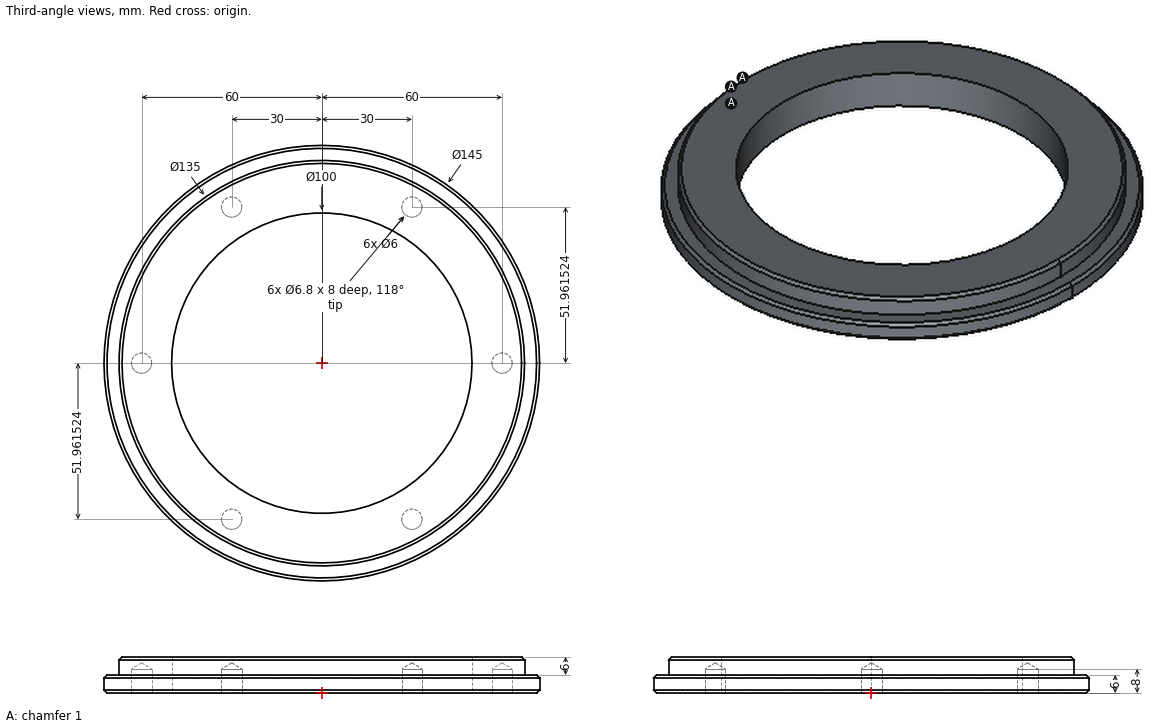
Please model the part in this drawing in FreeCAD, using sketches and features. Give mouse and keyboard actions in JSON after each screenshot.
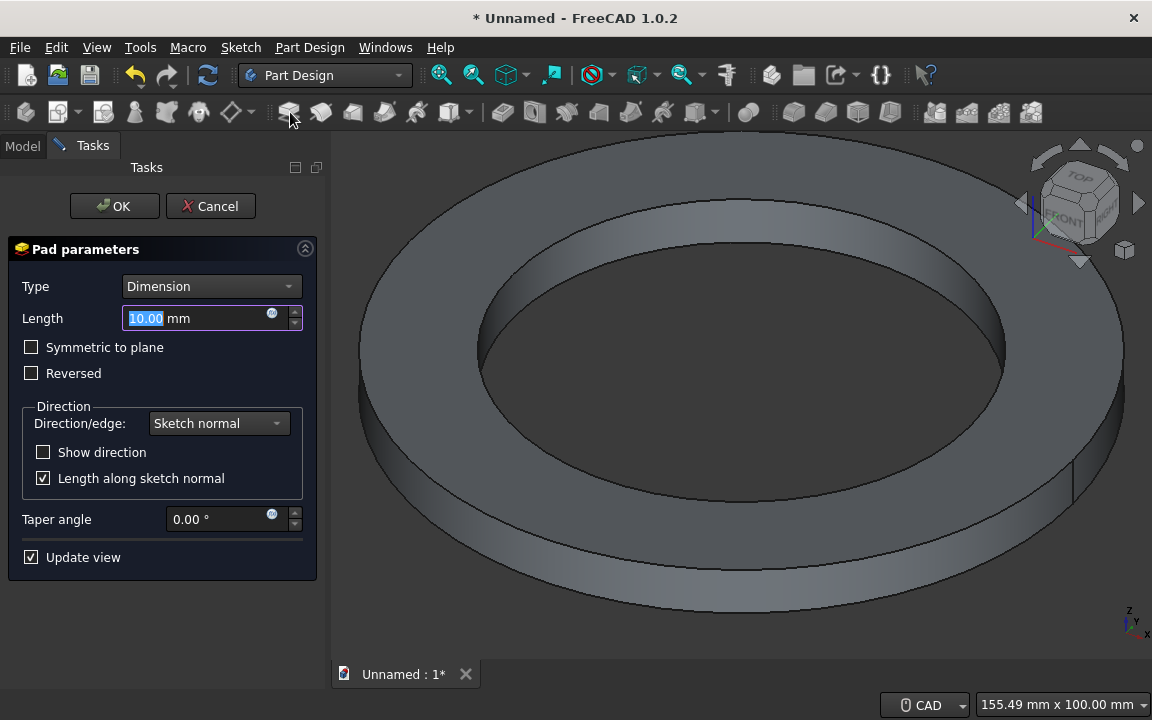
{"action": "type", "text": "6"}
{"action": "key", "text": "Tab"}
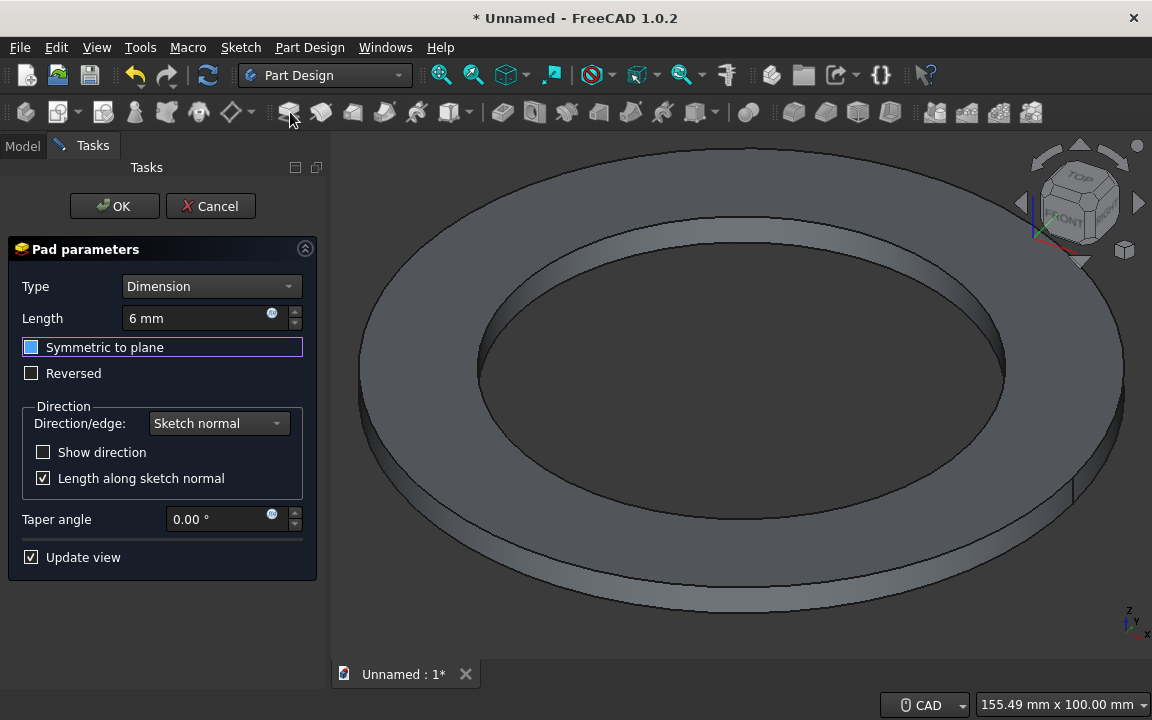
{"action": "left_click", "coordinate": [115, 206]}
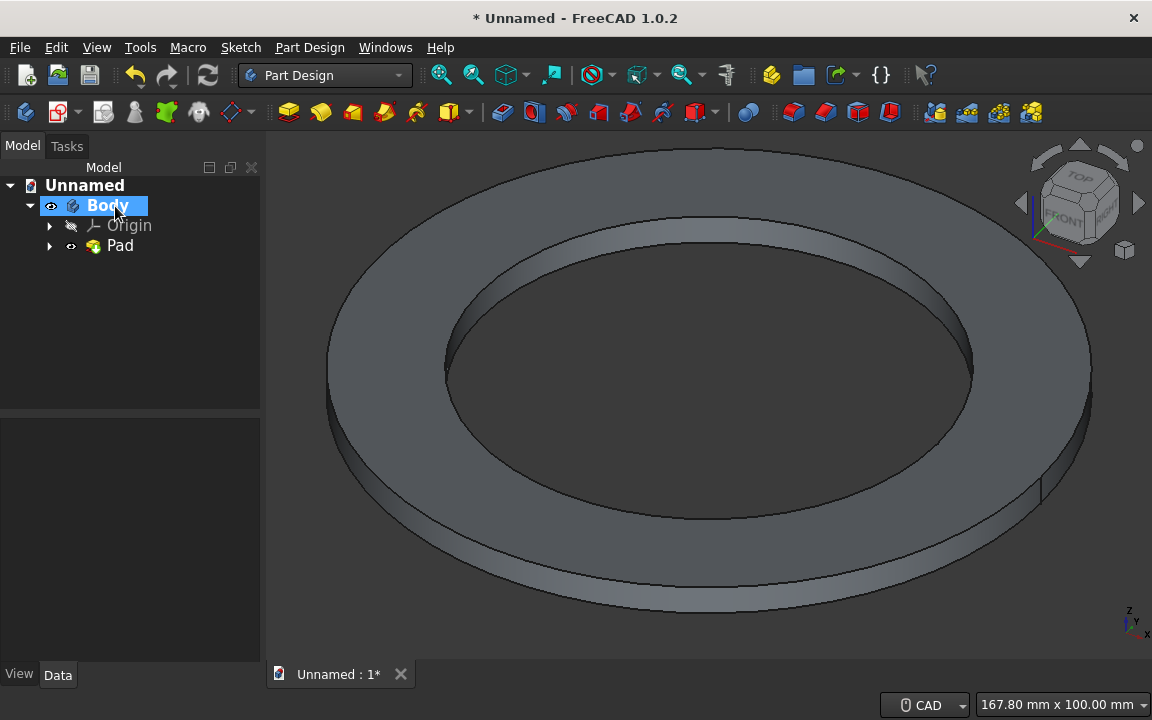
{"action": "left_click", "coordinate": [442, 76]}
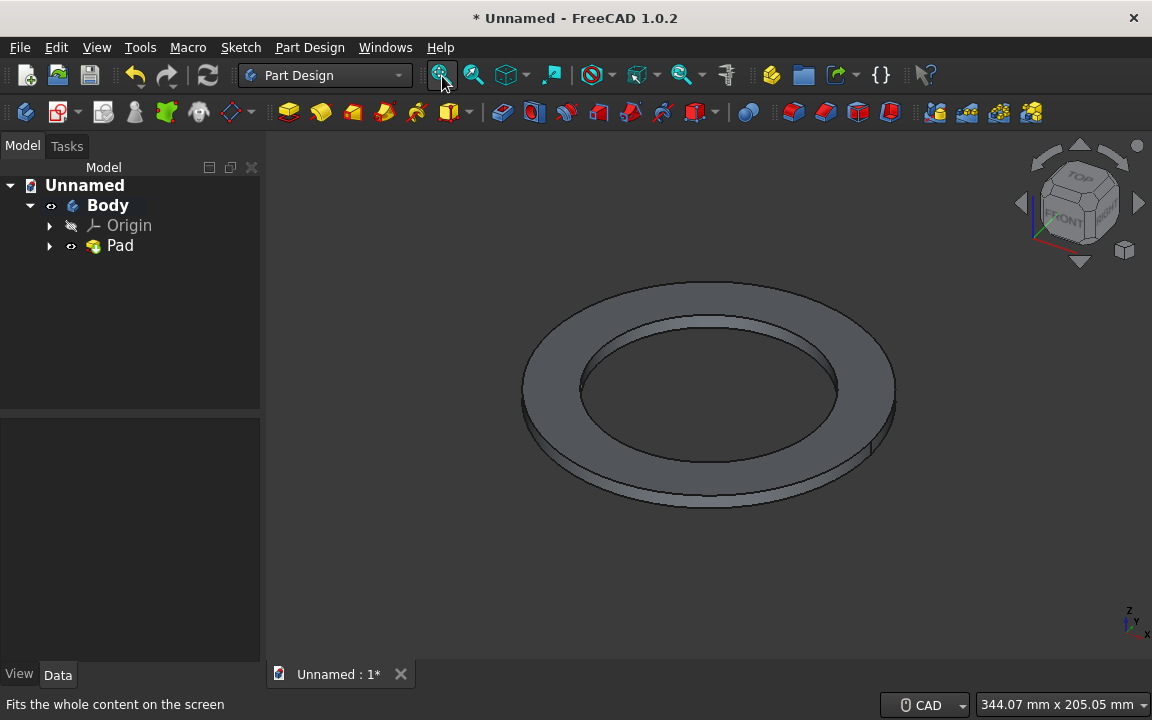
{"action": "left_click", "coordinate": [847, 434]}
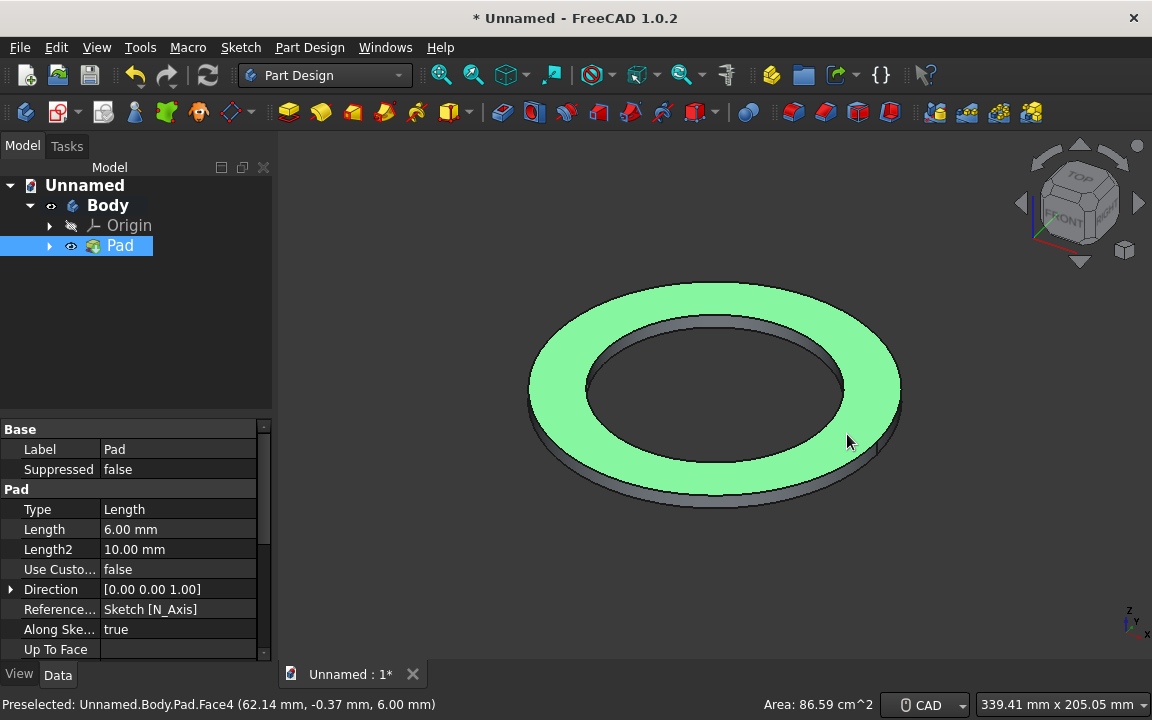
{"action": "left_click", "coordinate": [58, 112]}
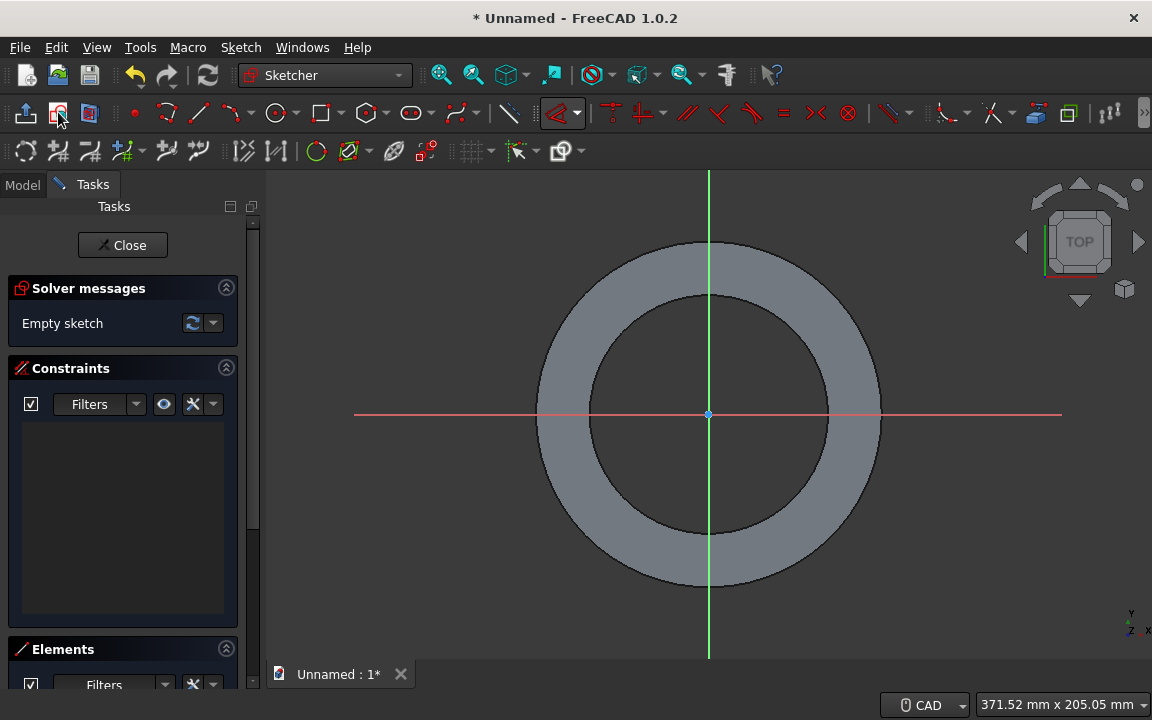
{"action": "left_click", "coordinate": [276, 114]}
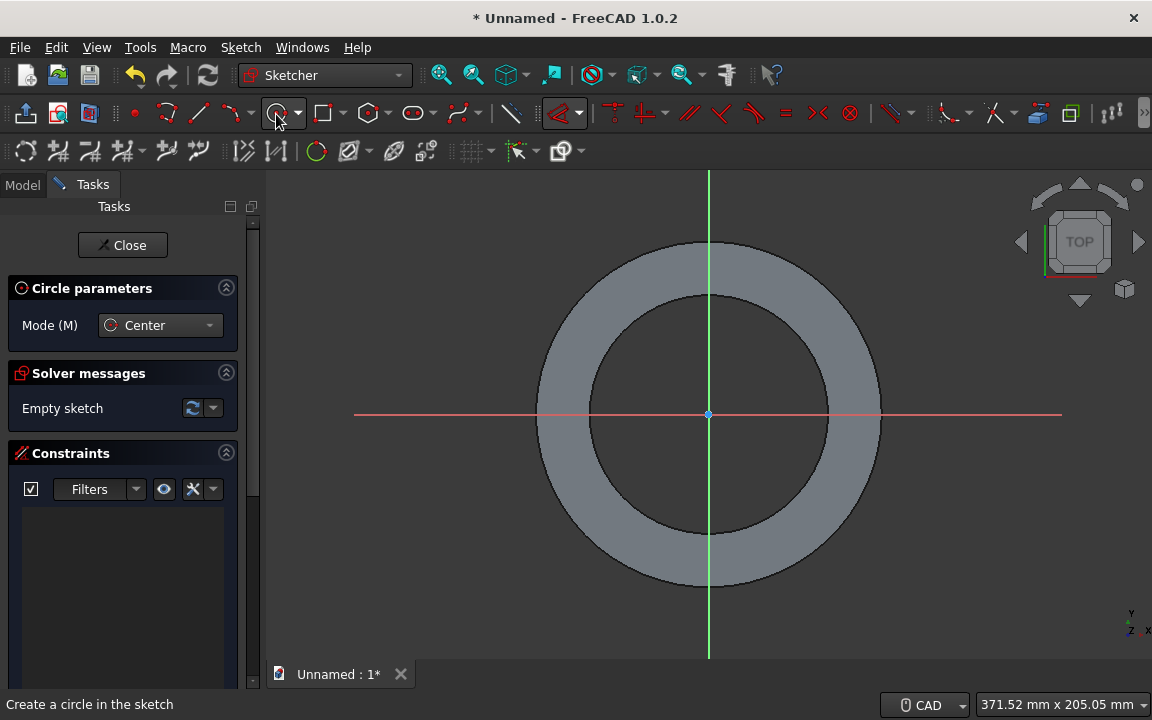
{"action": "left_click", "coordinate": [709, 414]}
{"action": "mouse_move", "coordinate": [823, 301]}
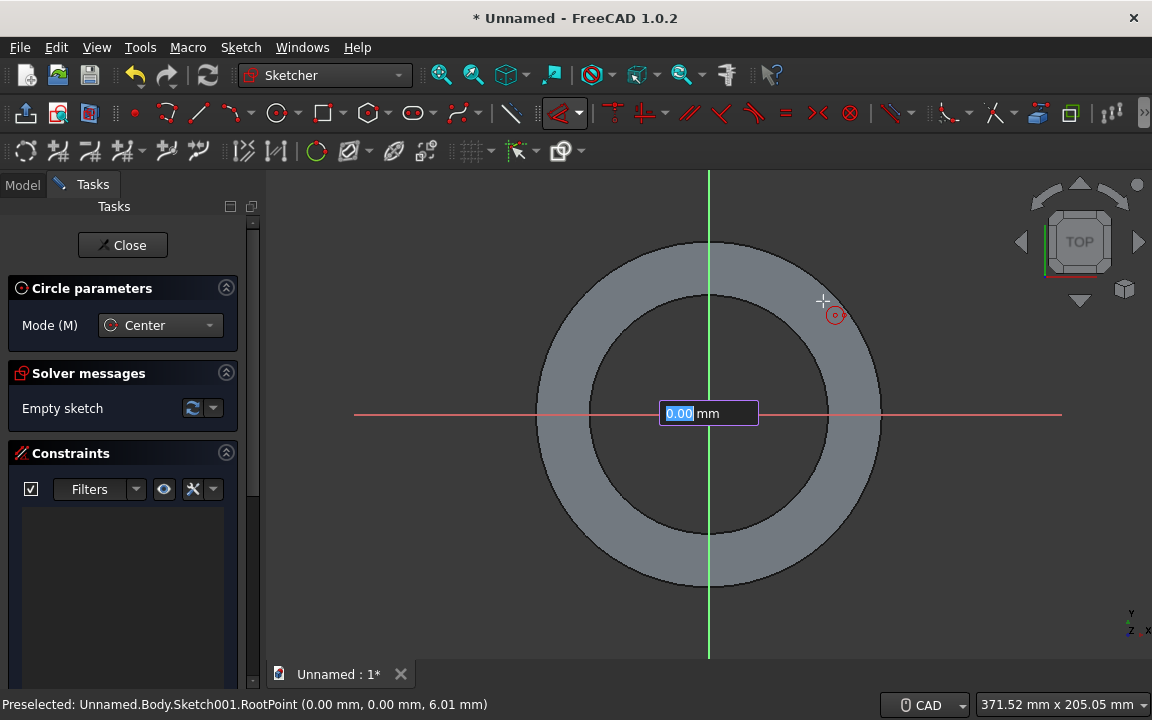
{"action": "type", "text": "135"}
{"action": "key", "text": "Return"}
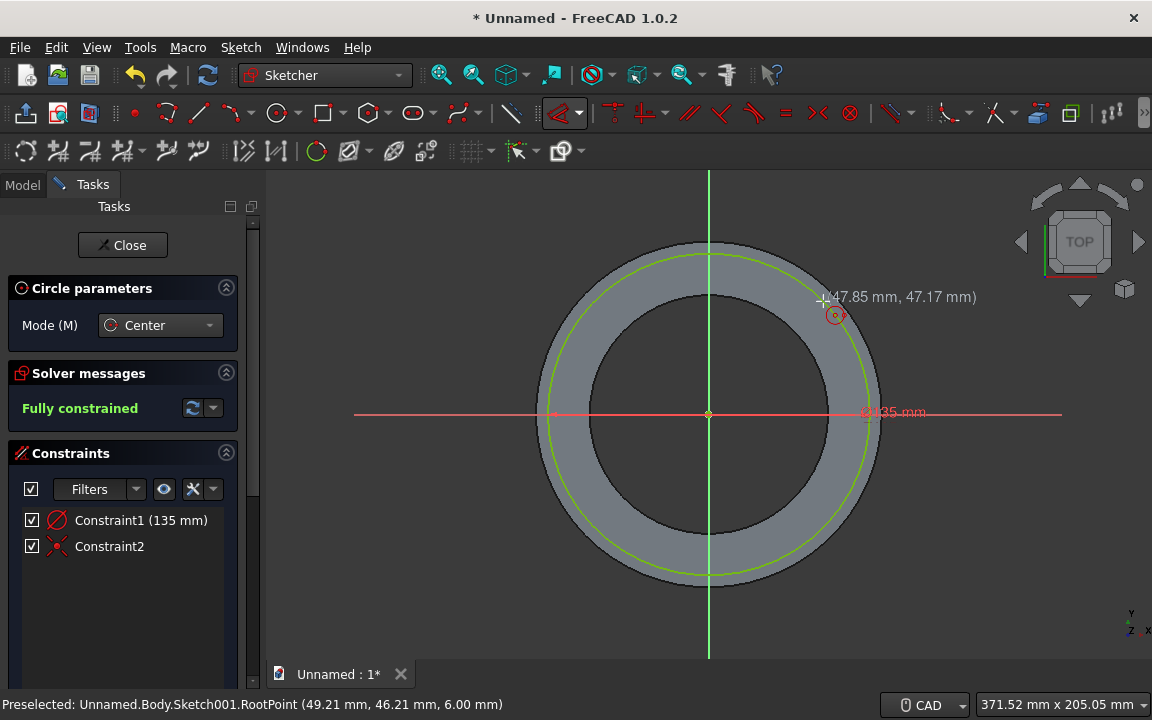
{"action": "left_click", "coordinate": [709, 414]}
{"action": "mouse_move", "coordinate": [793, 330]}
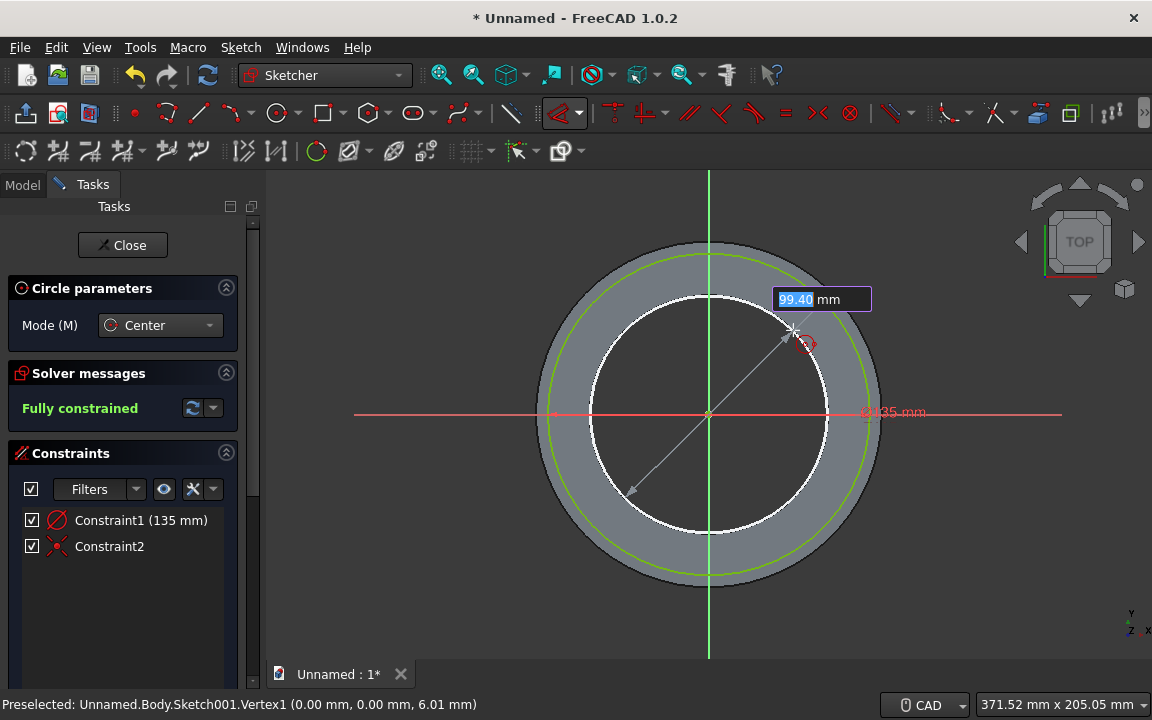
{"action": "type", "text": "100"}
{"action": "key", "text": "Return"}
{"action": "key", "text": "Escape"}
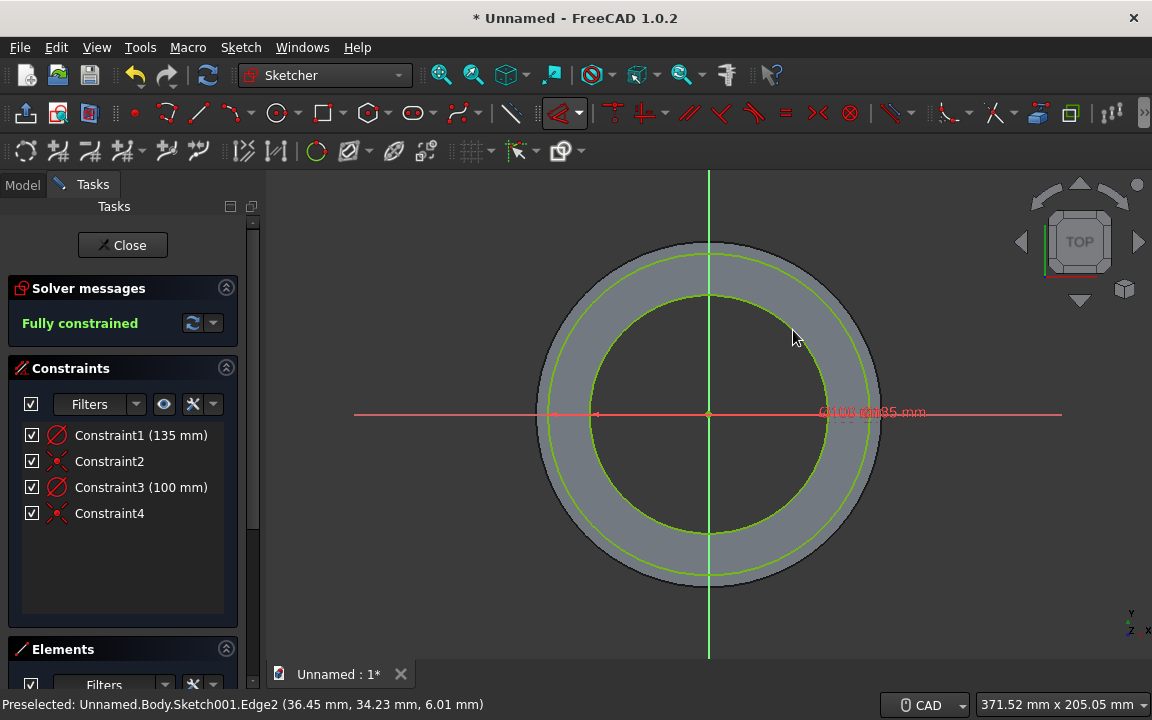
{"action": "left_click", "coordinate": [123, 245]}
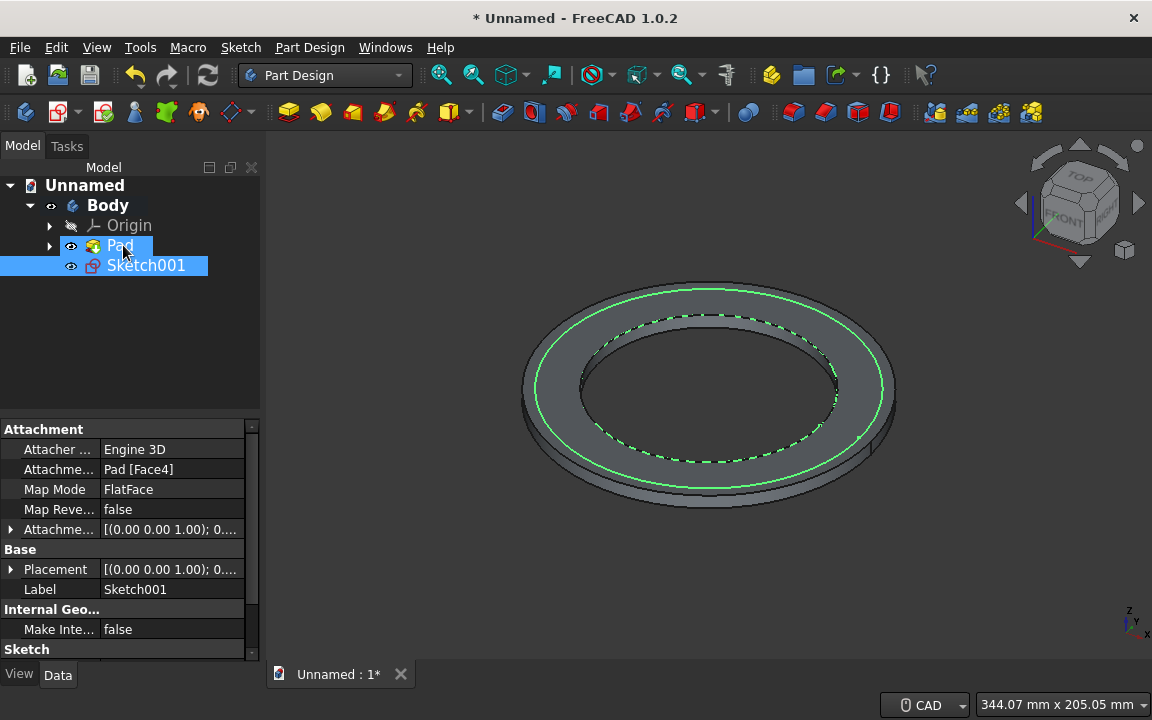
{"action": "left_click", "coordinate": [290, 112]}